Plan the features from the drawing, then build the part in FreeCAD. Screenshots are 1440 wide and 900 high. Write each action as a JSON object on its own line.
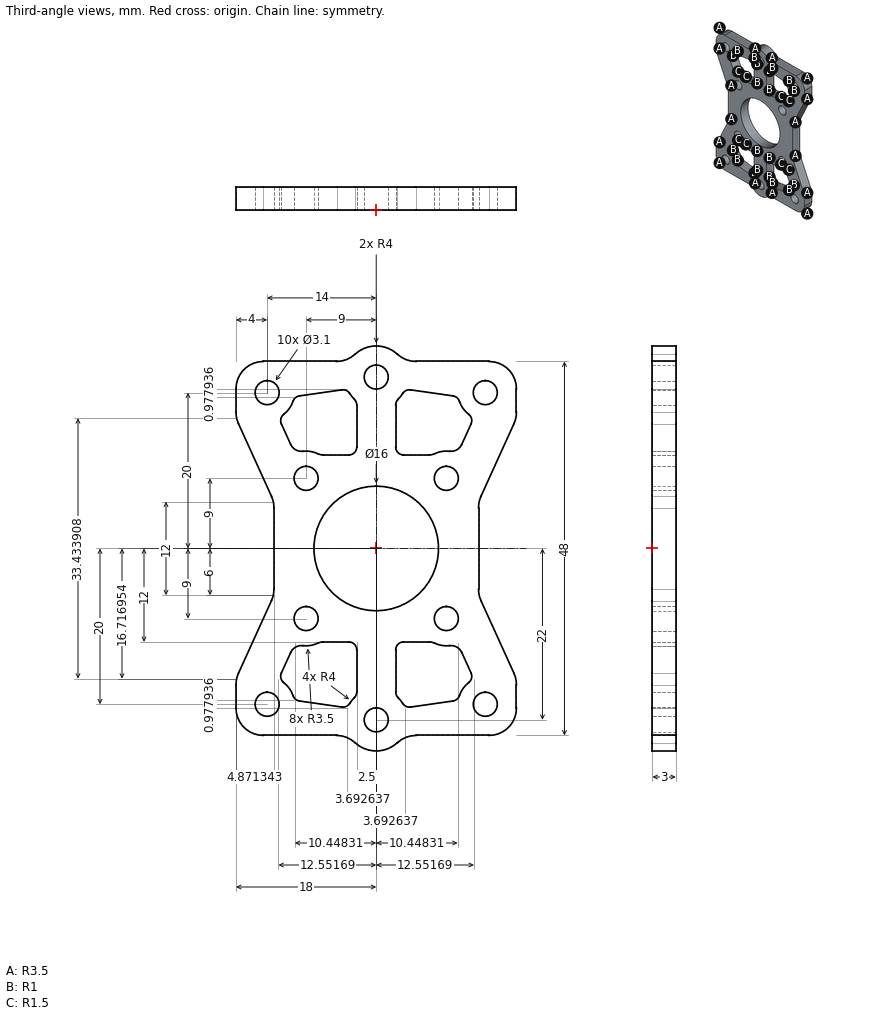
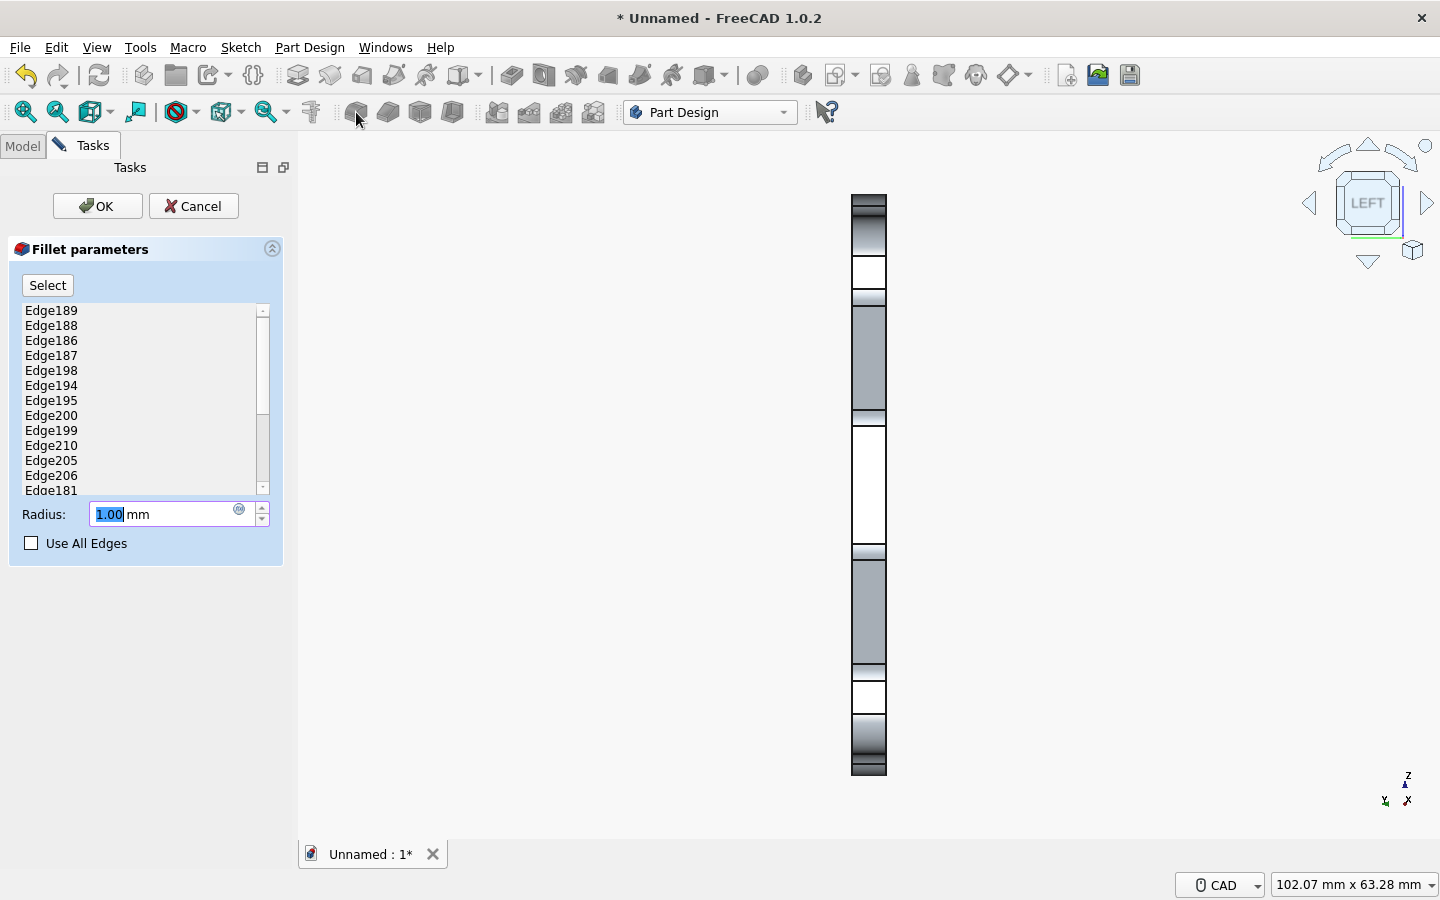
{"action": "type", "text": "1"}
{"action": "key", "text": "Tab"}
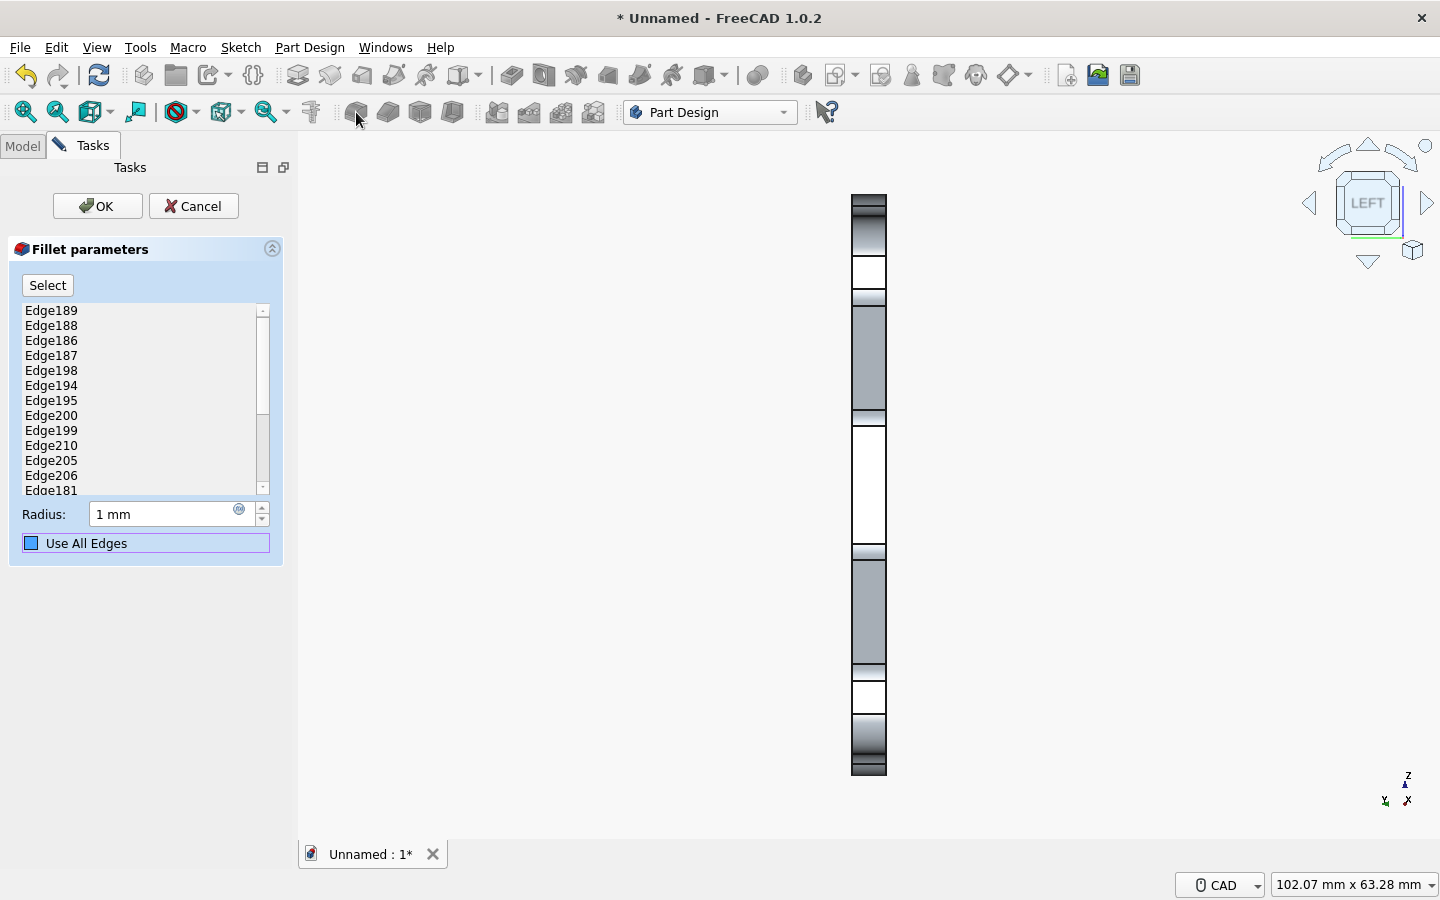
{"action": "left_click", "coordinate": [98, 206]}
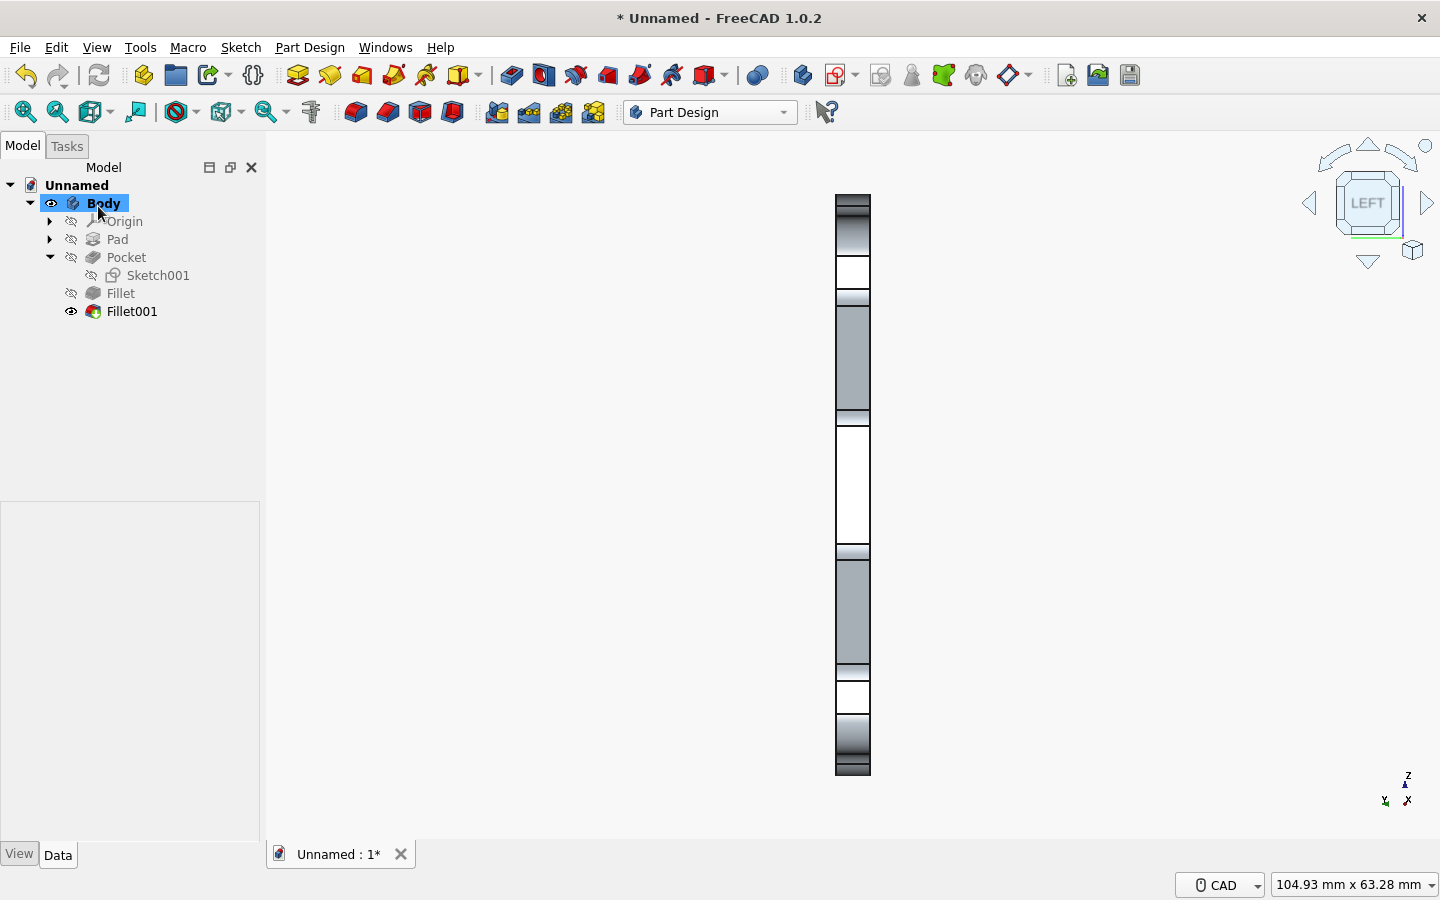
{"action": "key", "text": "0"}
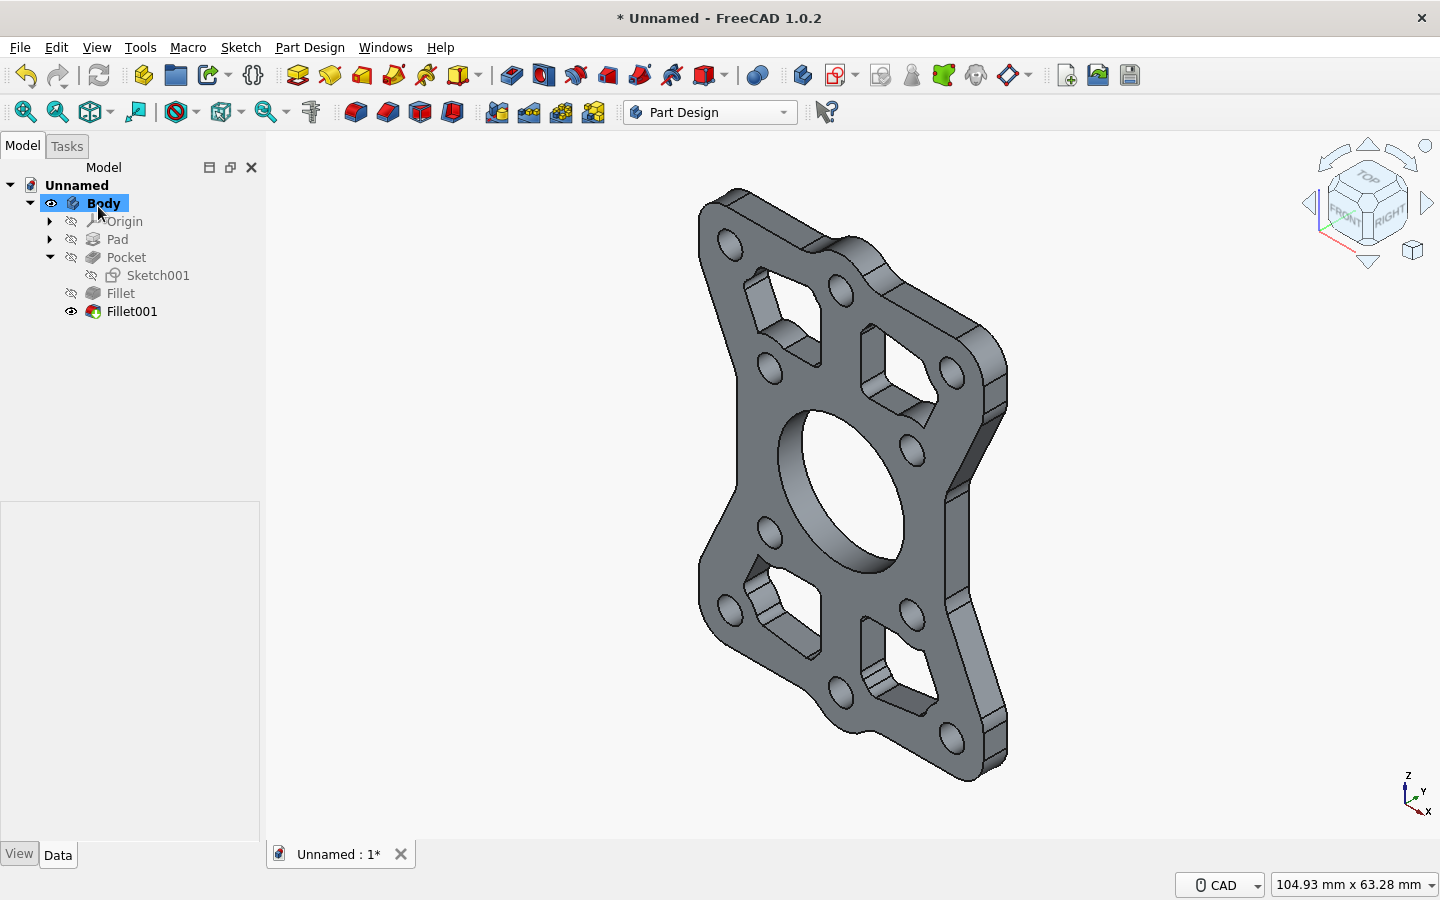
{"action": "key", "text": "2"}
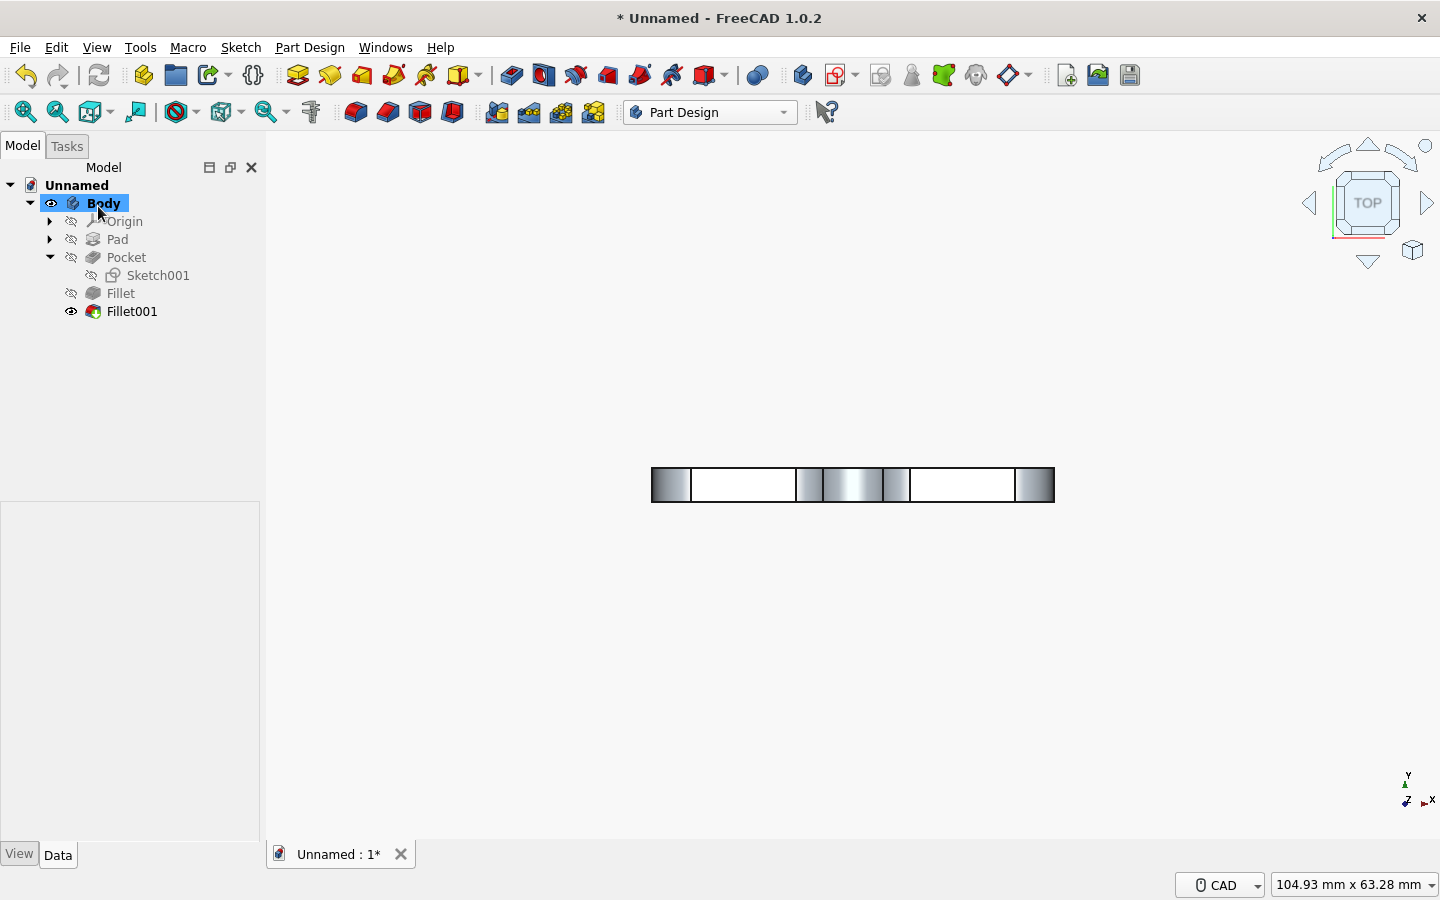
{"action": "key", "text": "v f"}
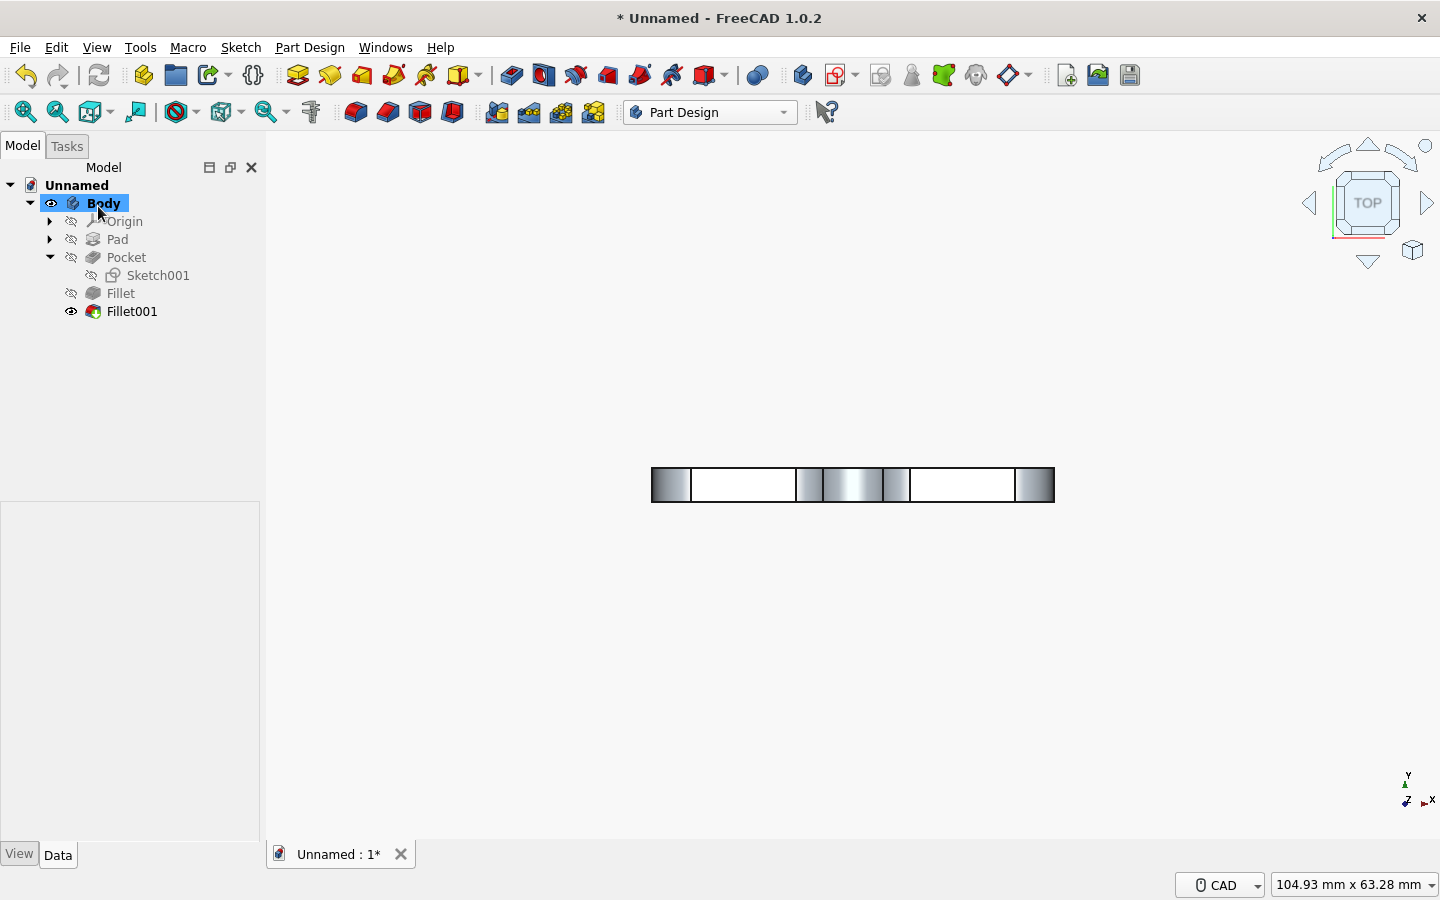
{"action": "key", "text": "1"}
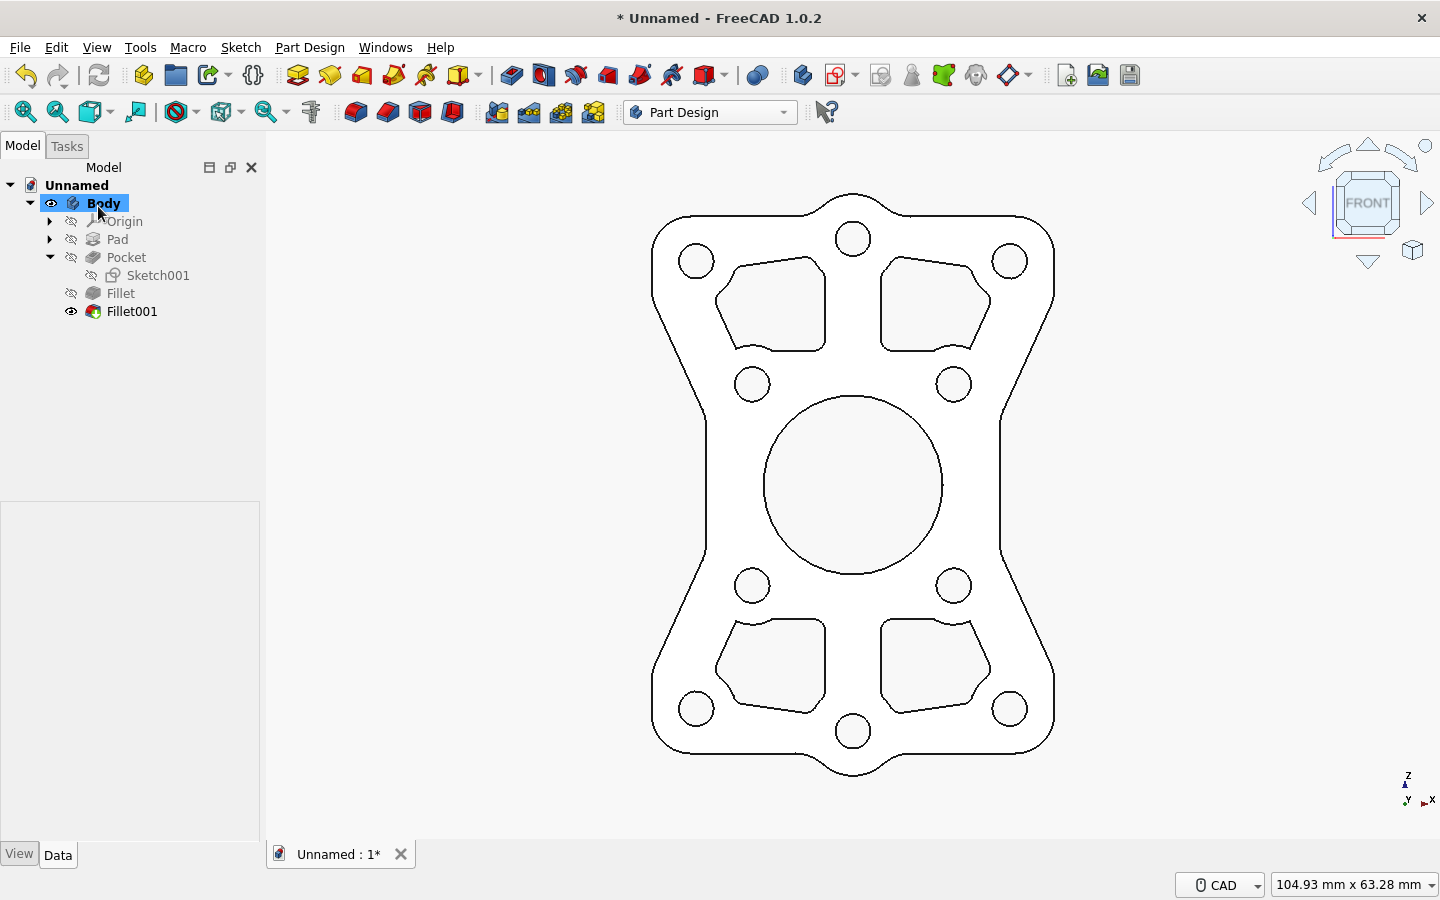
{"action": "key", "text": "3"}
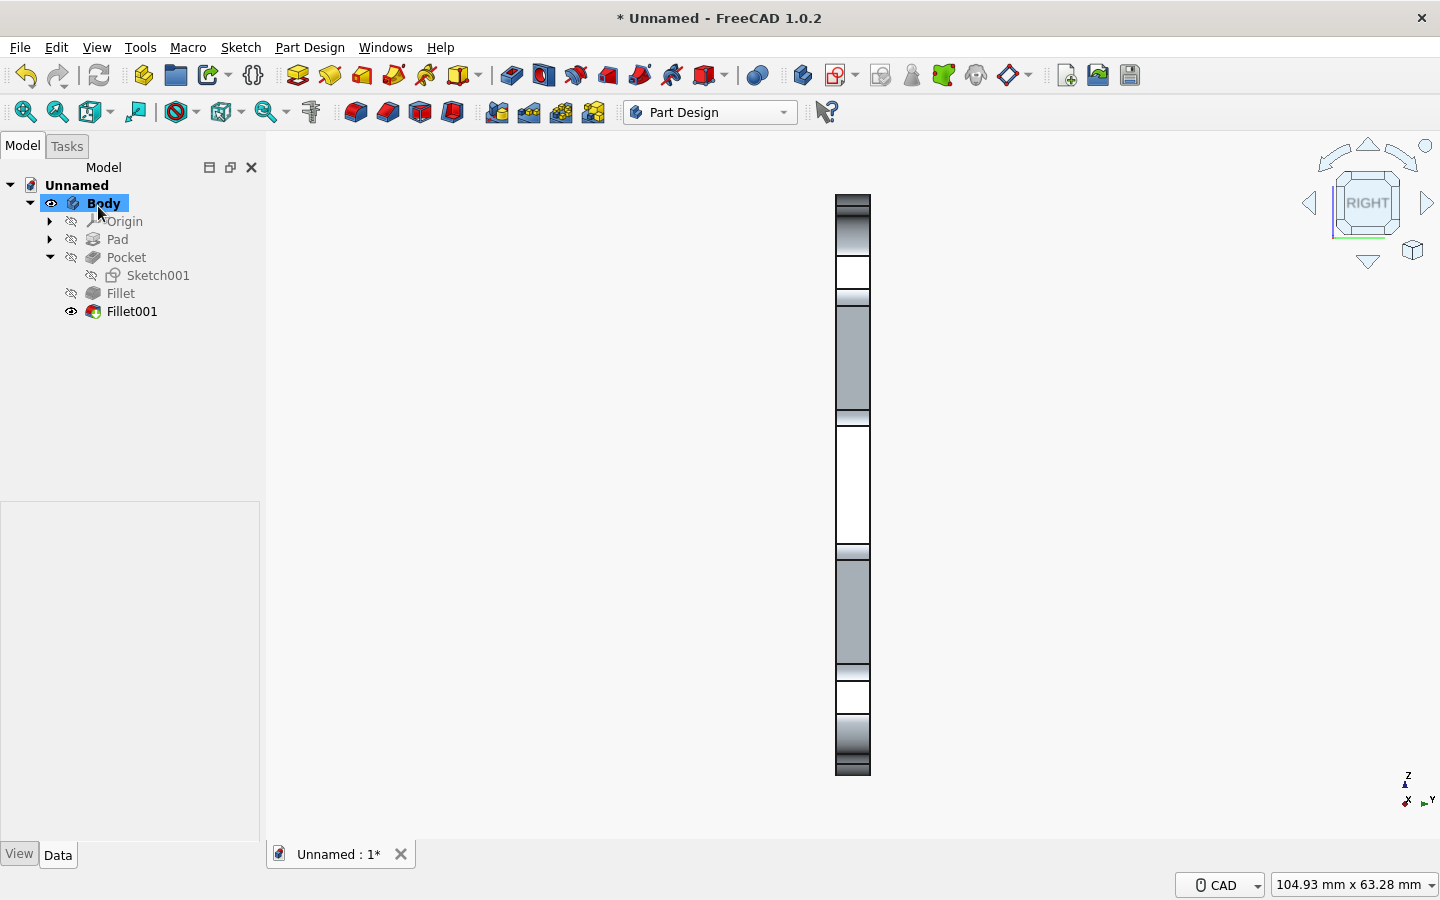
{"action": "key", "text": "5"}